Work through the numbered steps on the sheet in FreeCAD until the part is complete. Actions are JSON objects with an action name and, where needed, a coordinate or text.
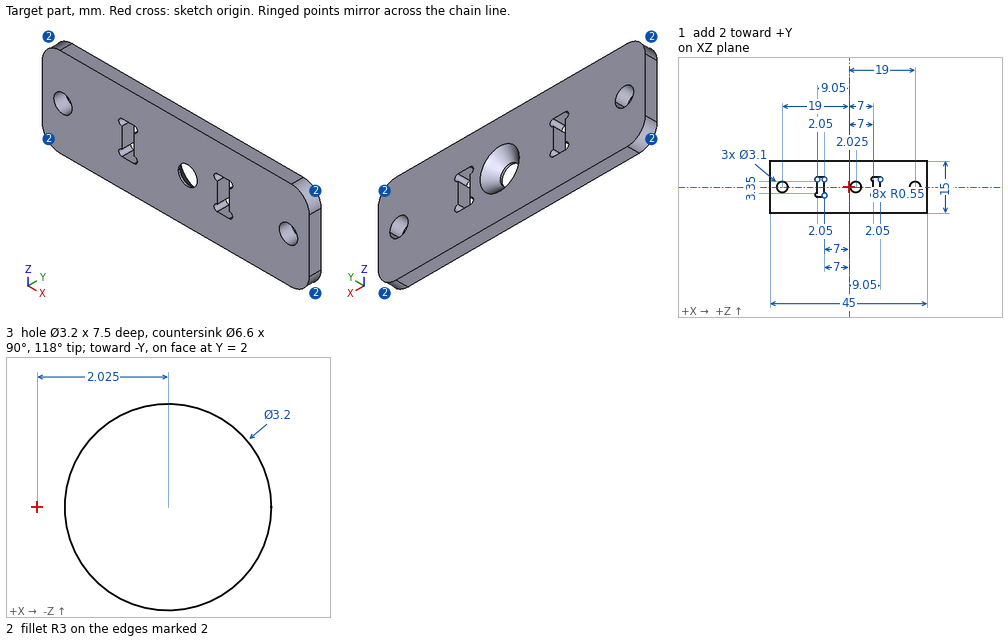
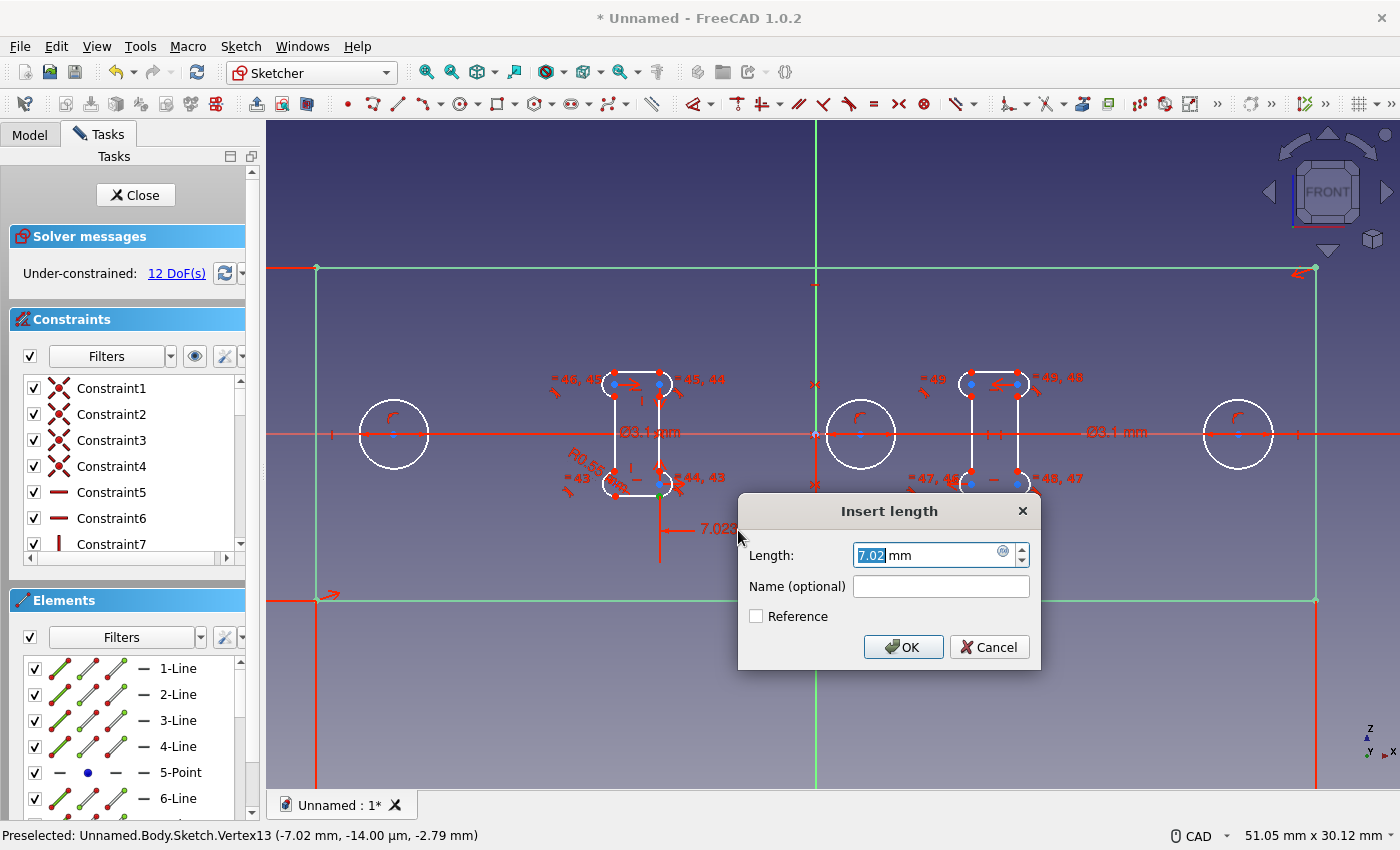
{"action": "type", "text": "7"}
{"action": "key", "text": "Return"}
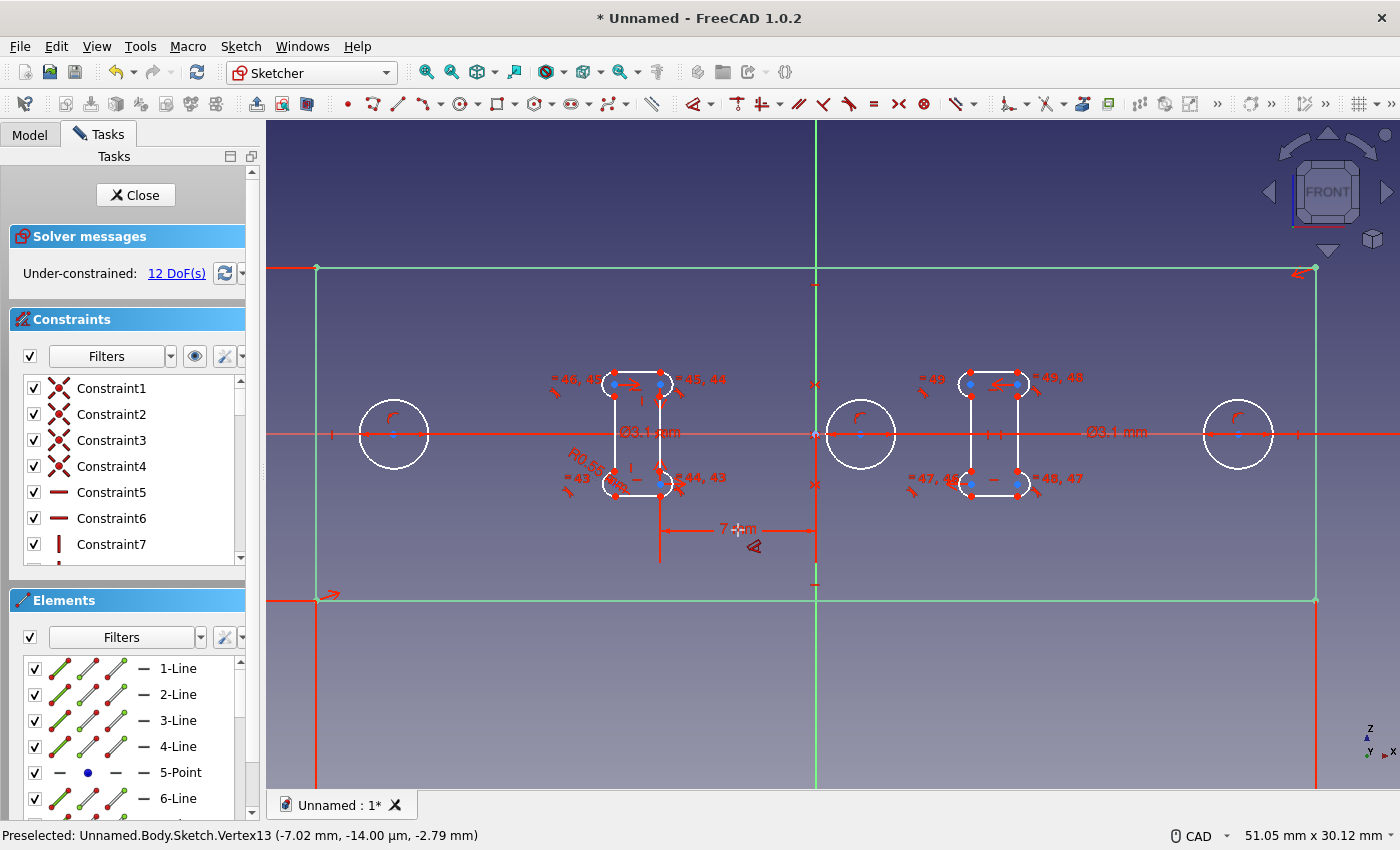
{"action": "left_click", "coordinate": [660, 472]}
{"action": "left_click", "coordinate": [738, 506]}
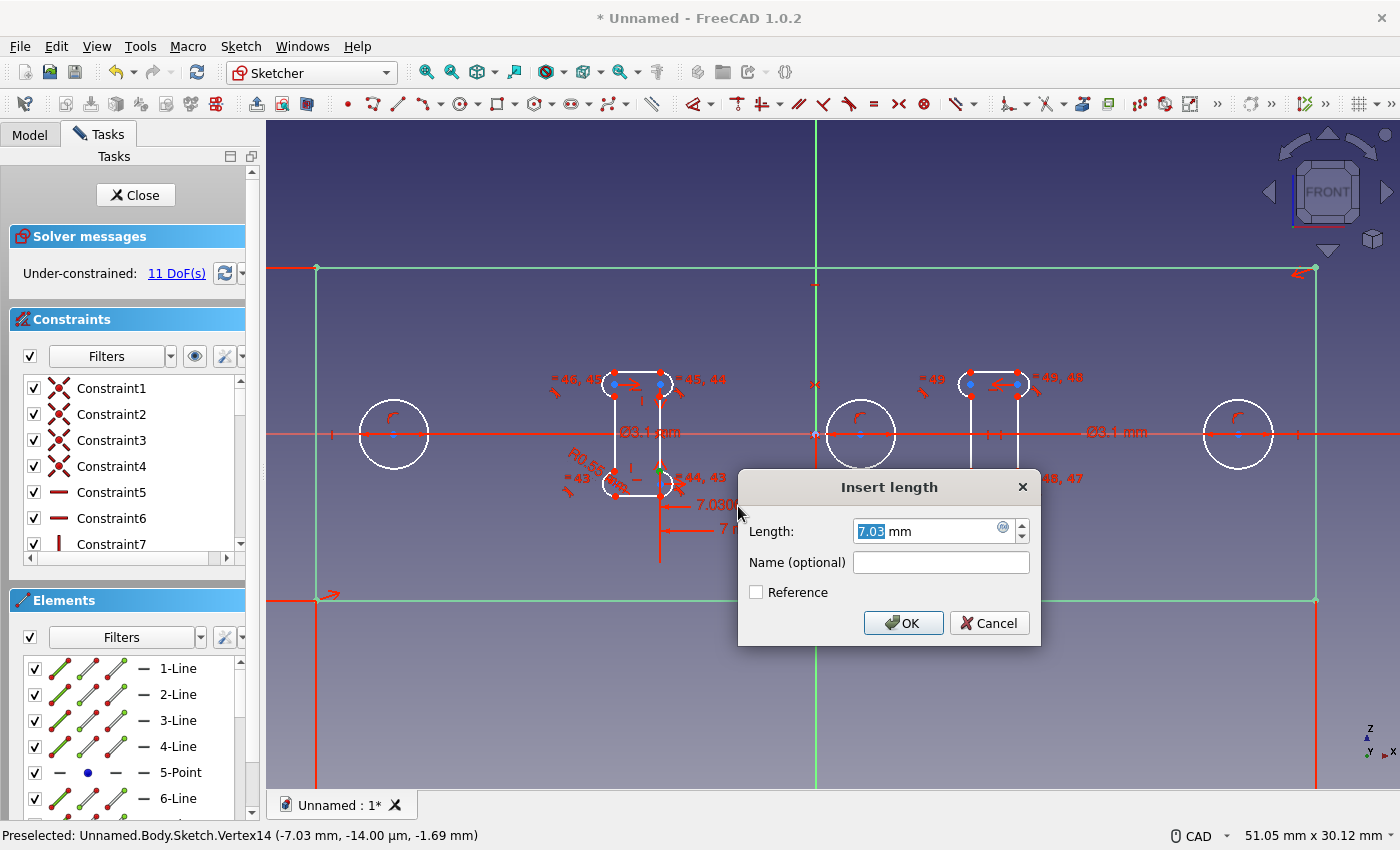
{"action": "type", "text": "7"}
{"action": "key", "text": "Return"}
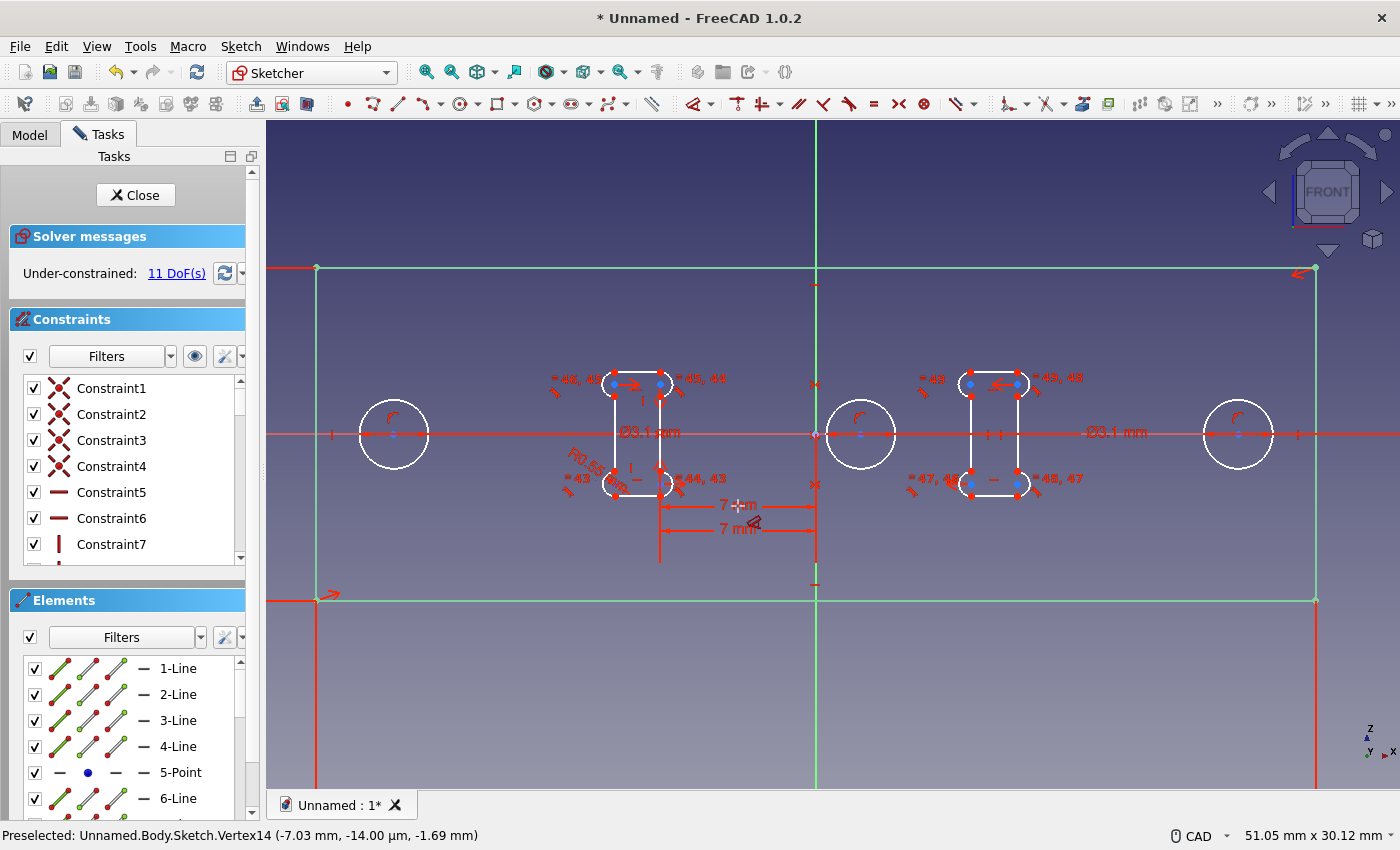
{"action": "left_click", "coordinate": [971, 397]}
{"action": "left_click", "coordinate": [894, 363]}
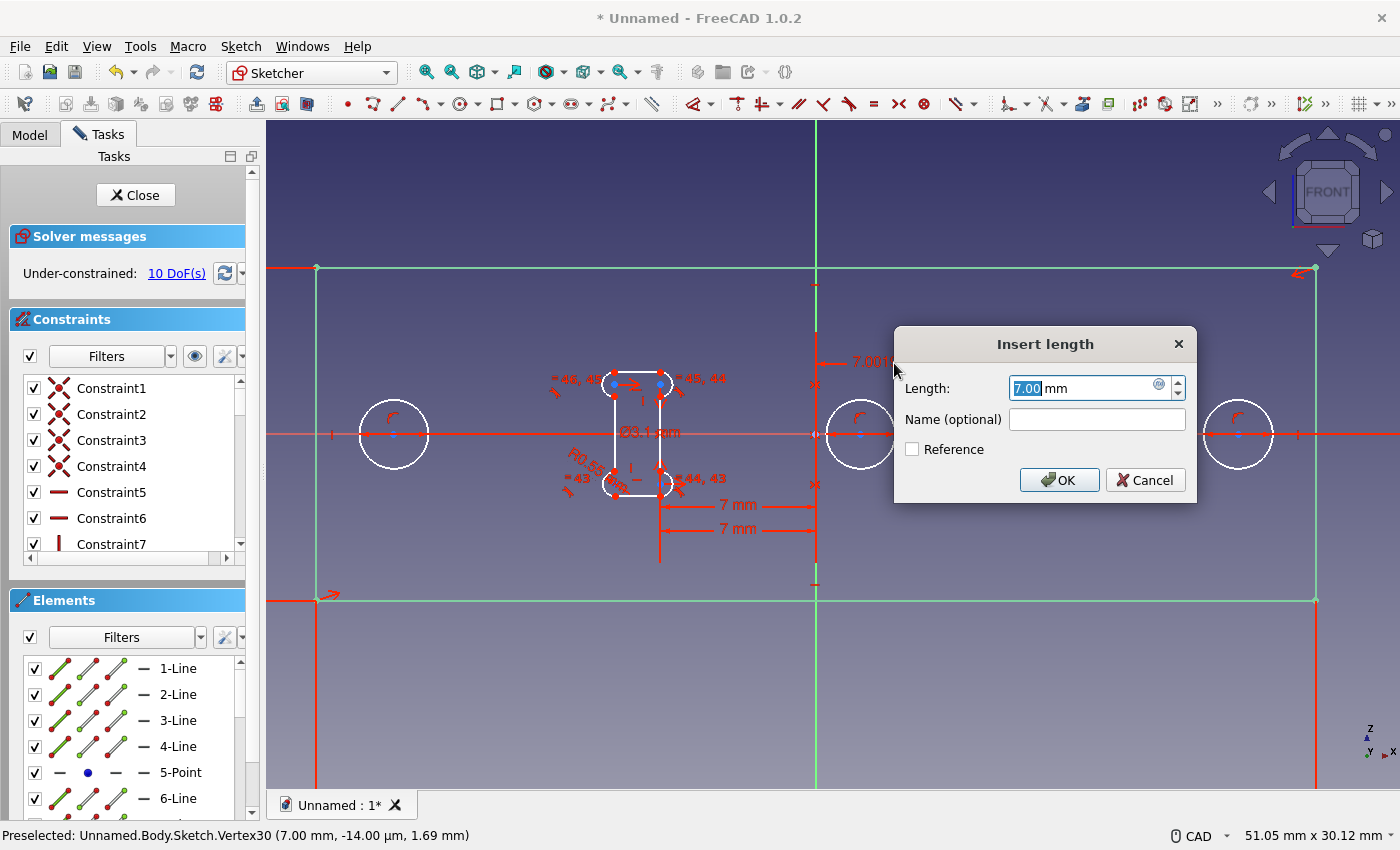
{"action": "type", "text": "7"}
{"action": "key", "text": "Return"}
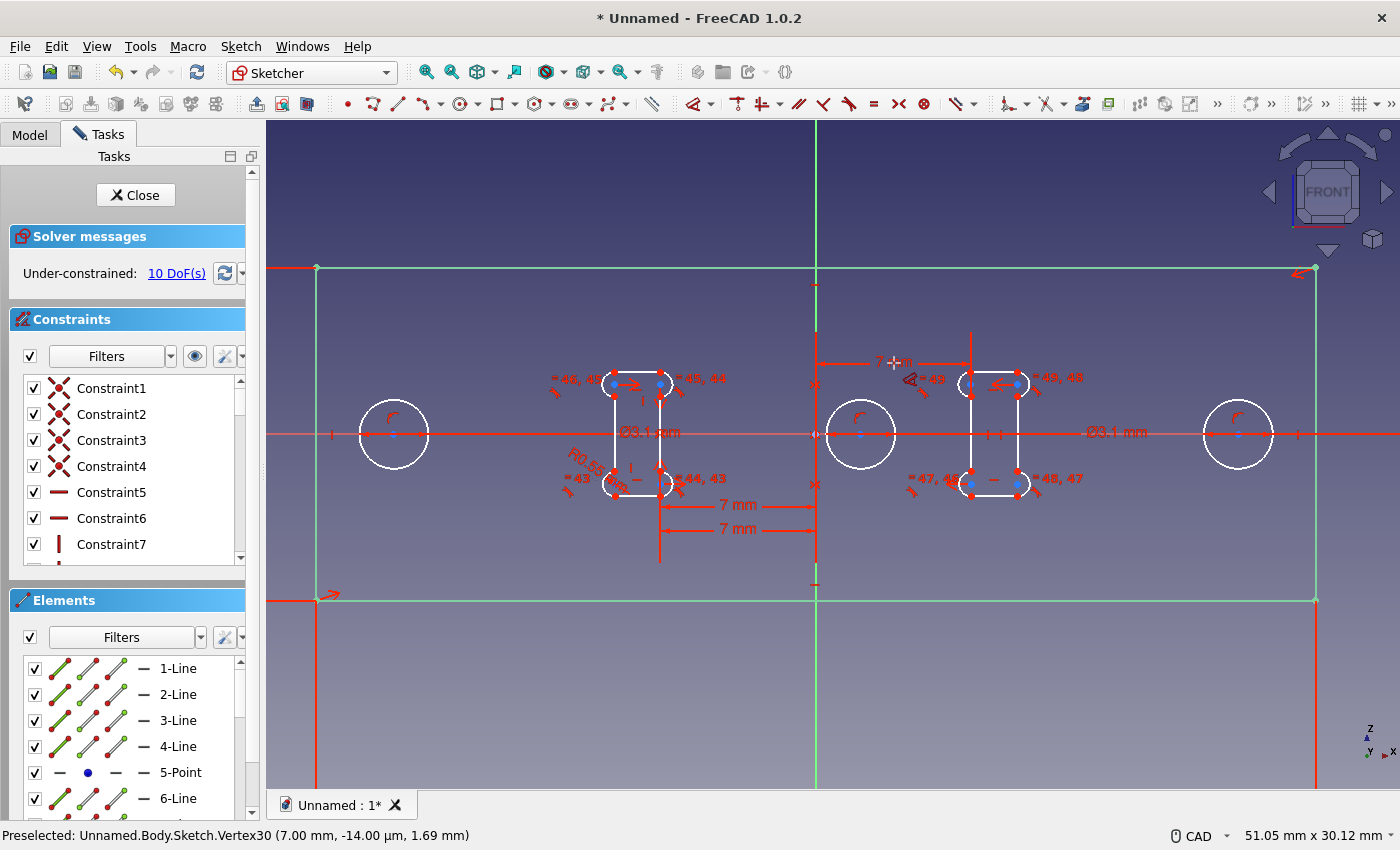
{"action": "left_click", "coordinate": [971, 372]}
{"action": "left_click", "coordinate": [893, 338]}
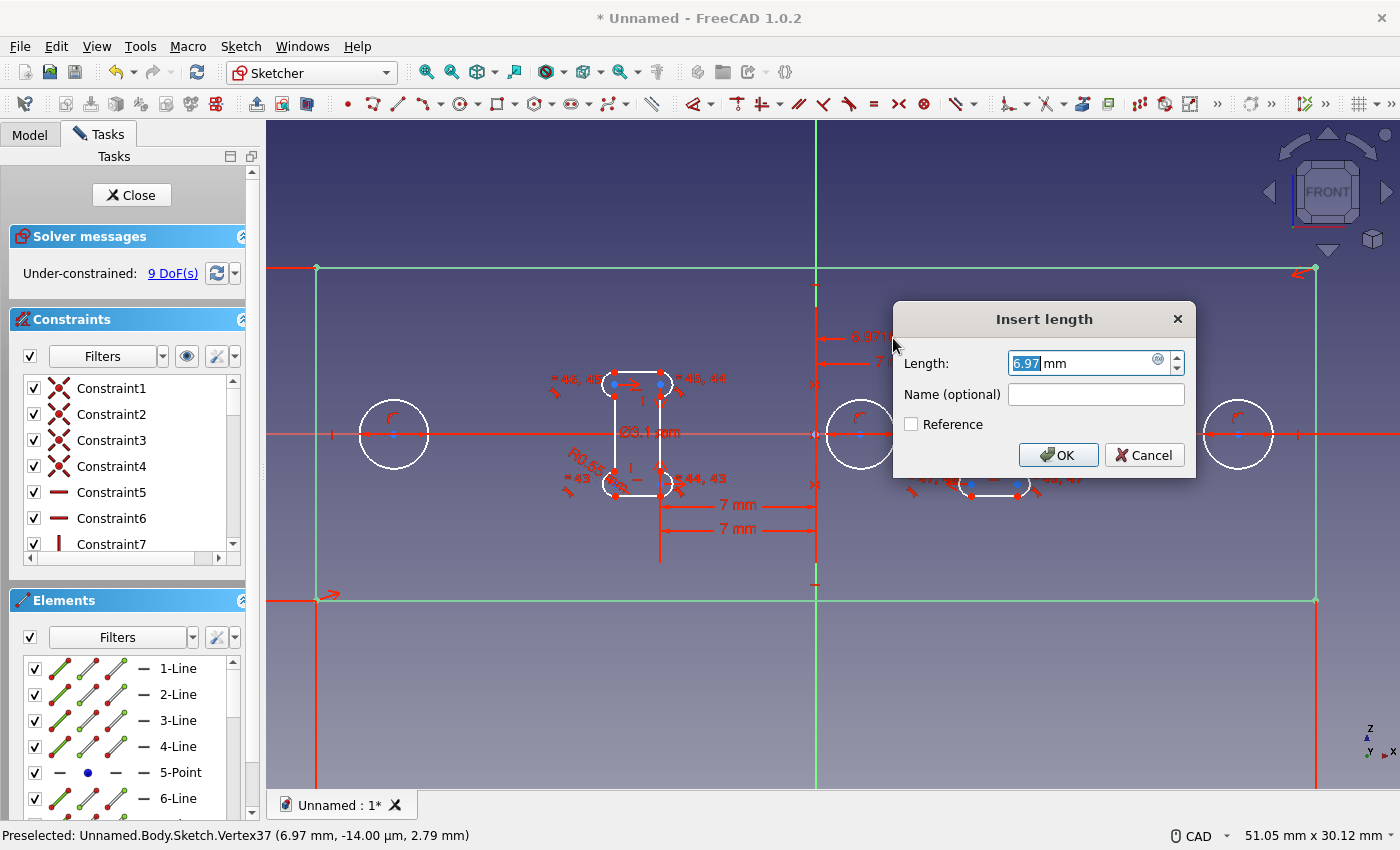
{"action": "type", "text": "7"}
{"action": "key", "text": "Return"}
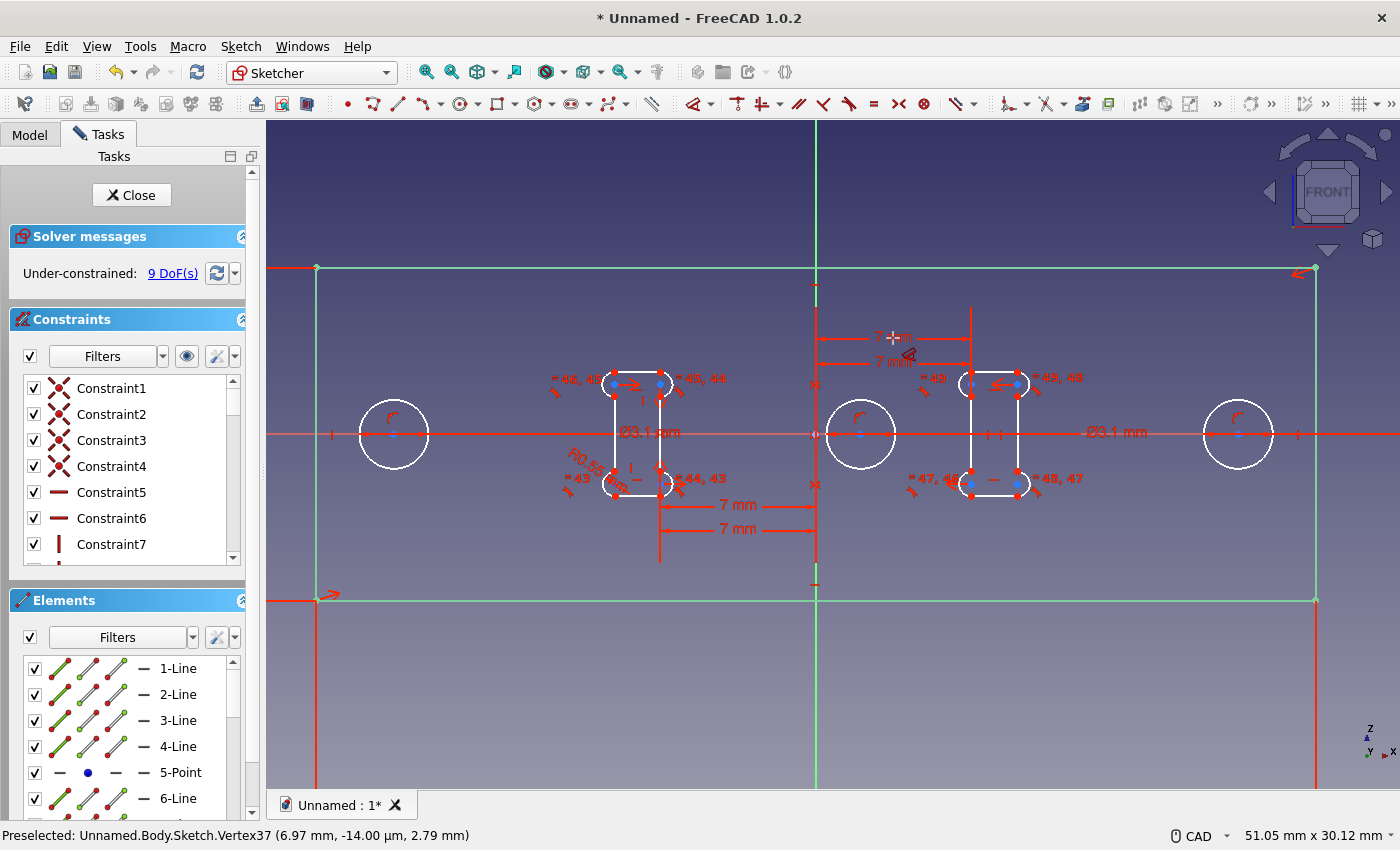
{"action": "left_click", "coordinate": [394, 434]}
{"action": "left_click", "coordinate": [508, 468]}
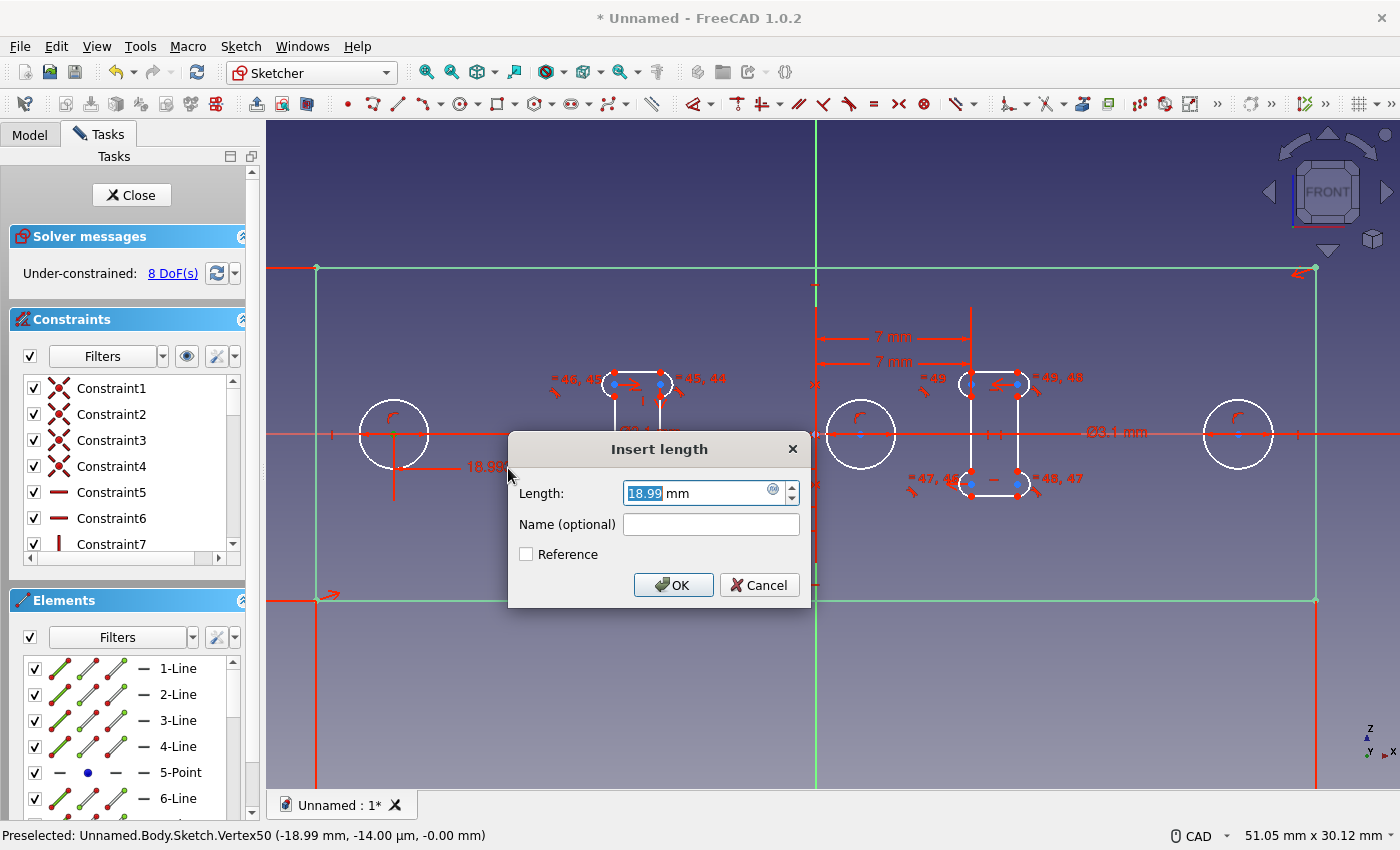
{"action": "type", "text": "19"}
{"action": "key", "text": "Return"}